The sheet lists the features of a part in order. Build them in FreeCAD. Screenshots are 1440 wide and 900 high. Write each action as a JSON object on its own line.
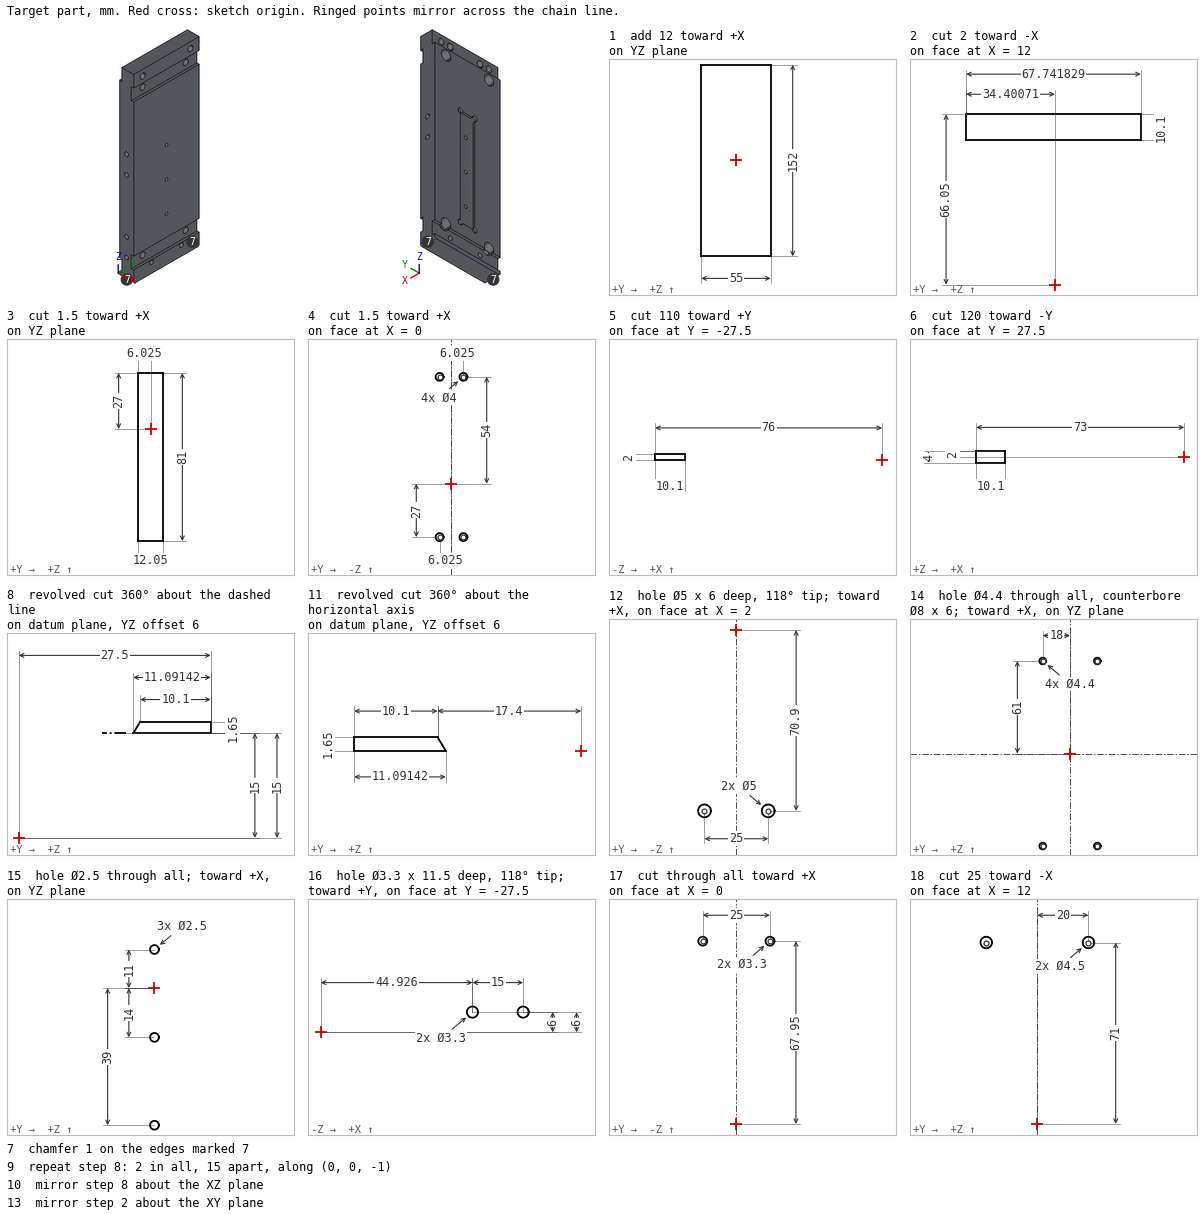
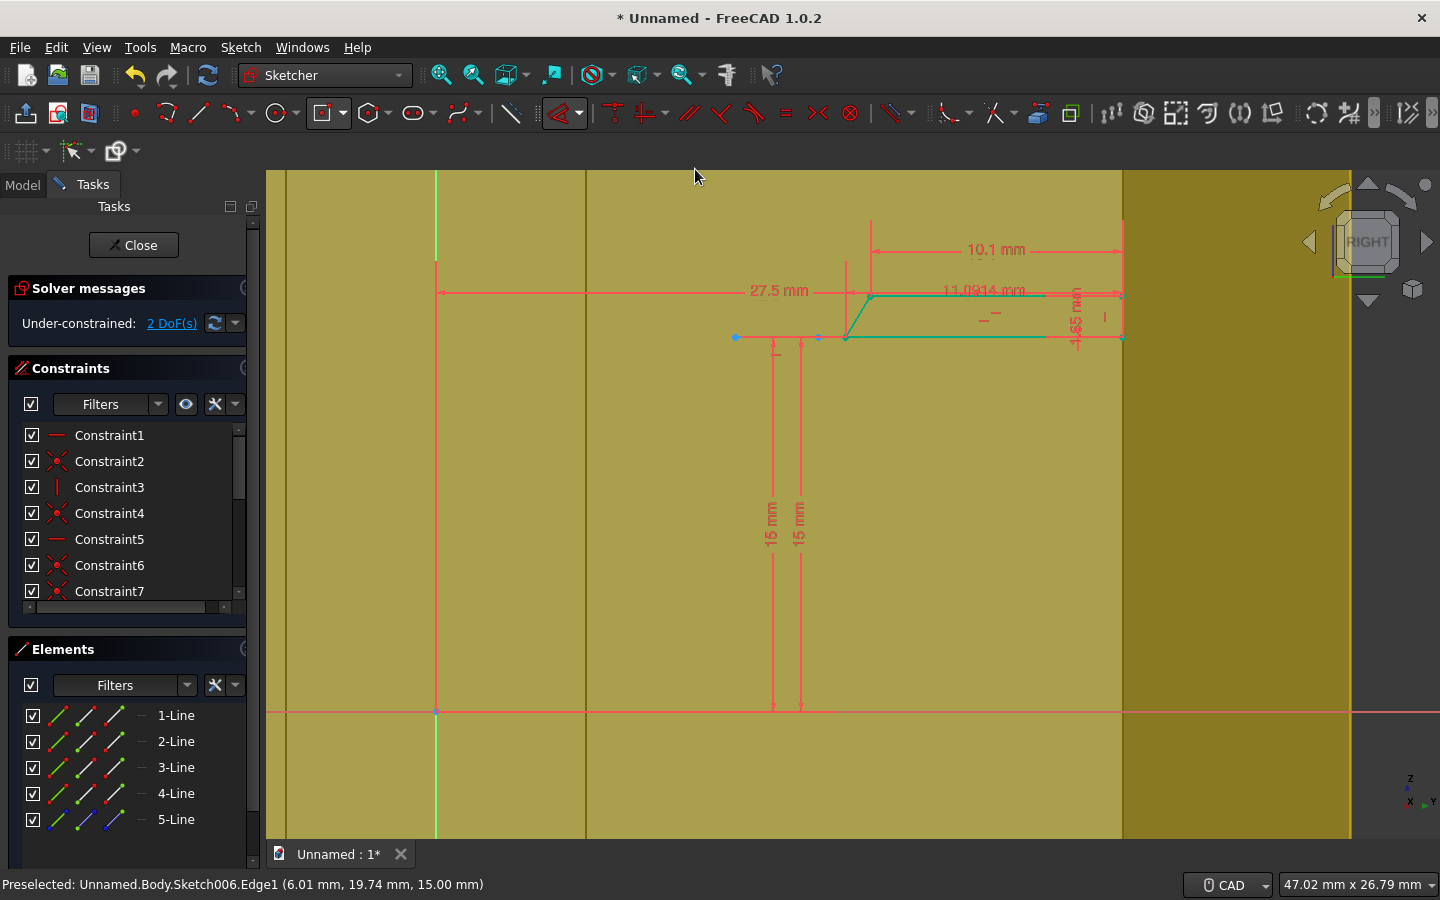
{"action": "left_click", "coordinate": [134, 245]}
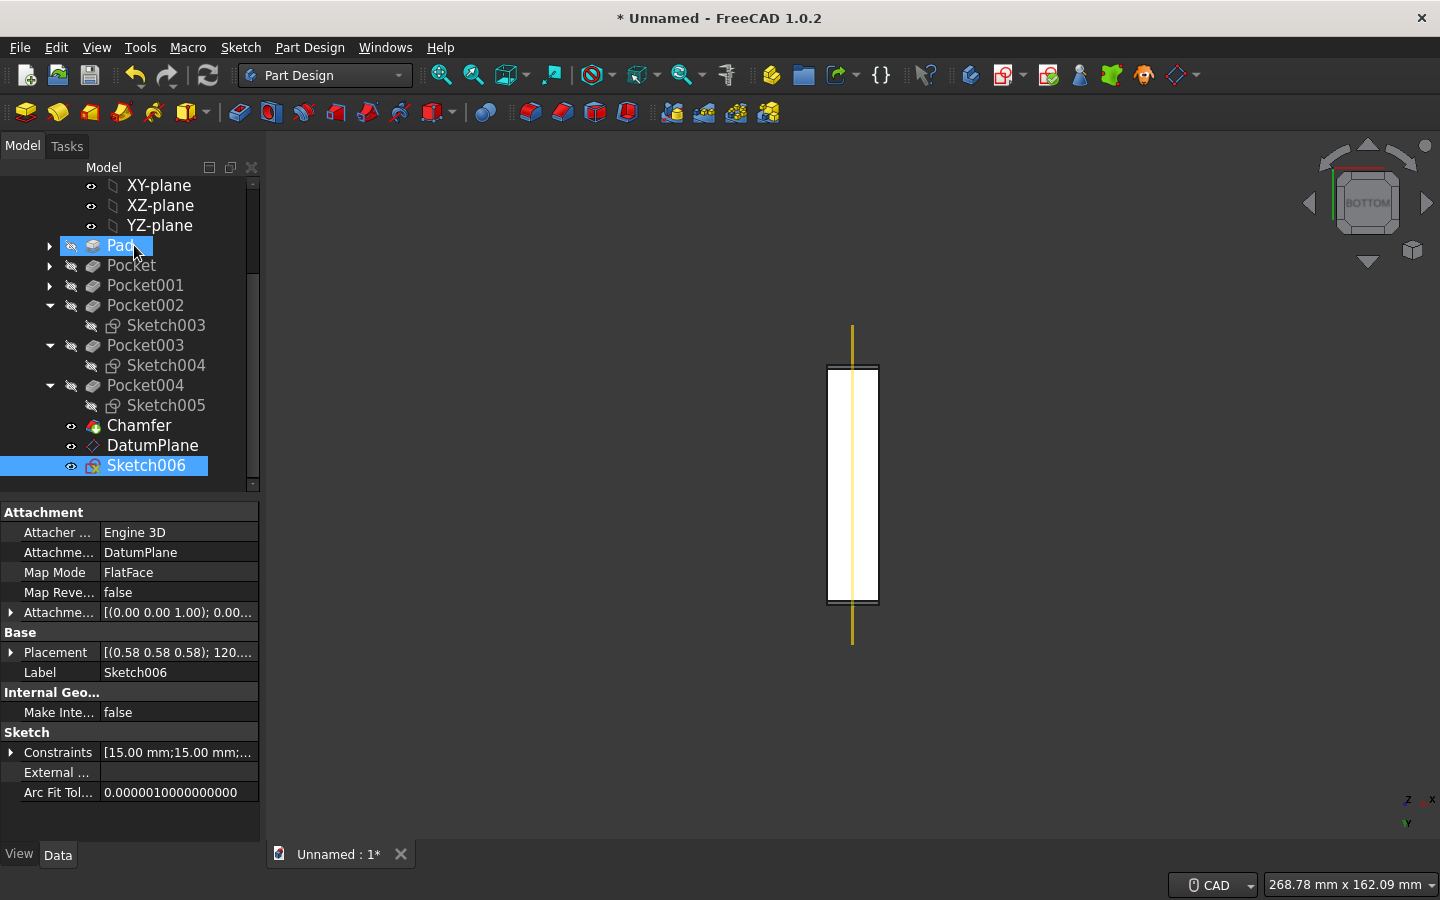
{"action": "left_click", "coordinate": [304, 112]}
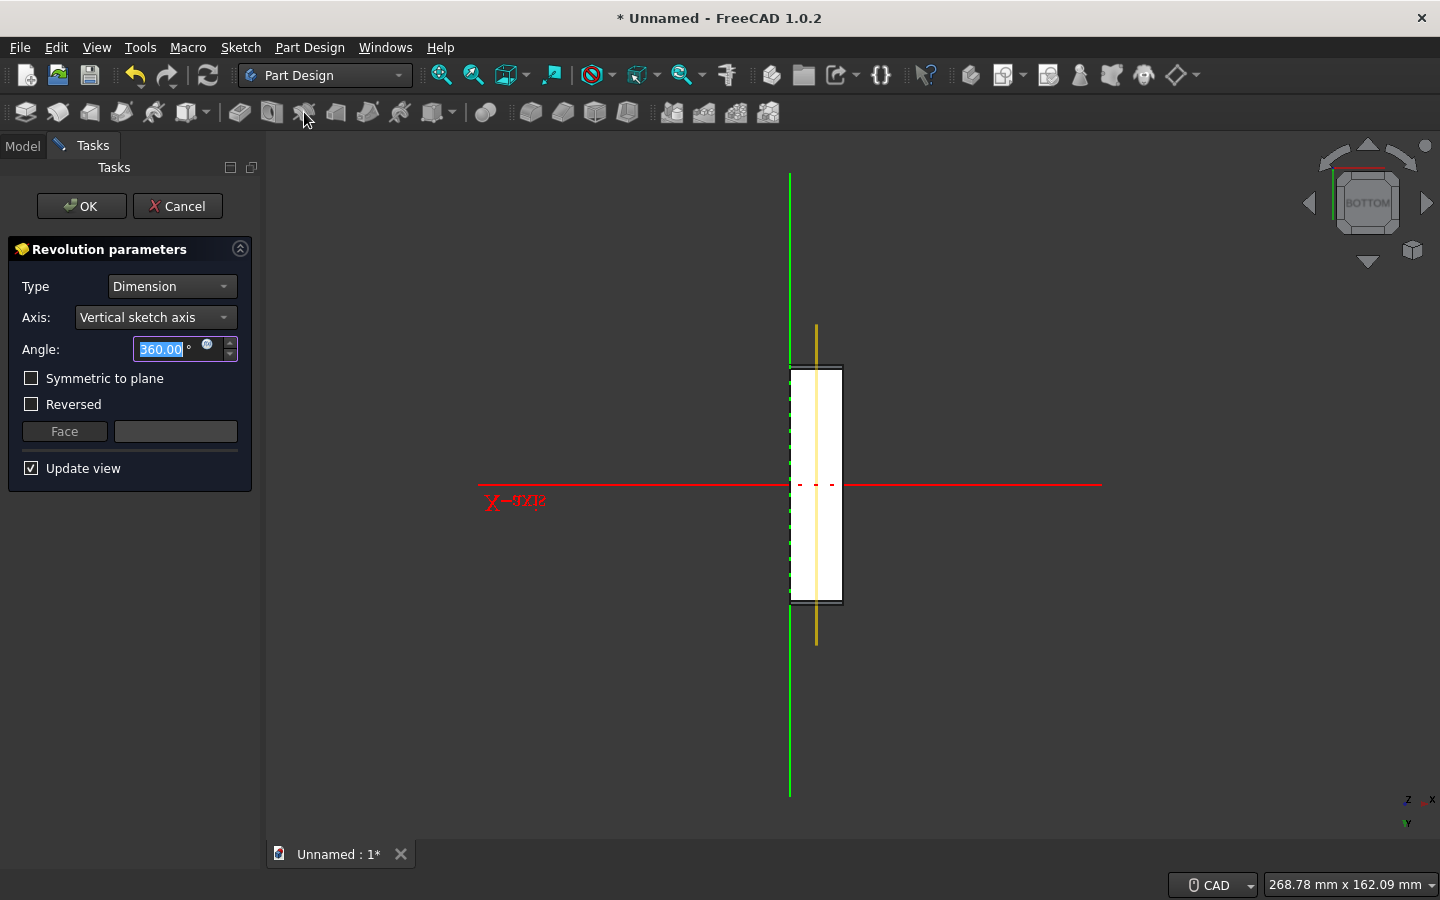
{"action": "left_click", "coordinate": [156, 318]}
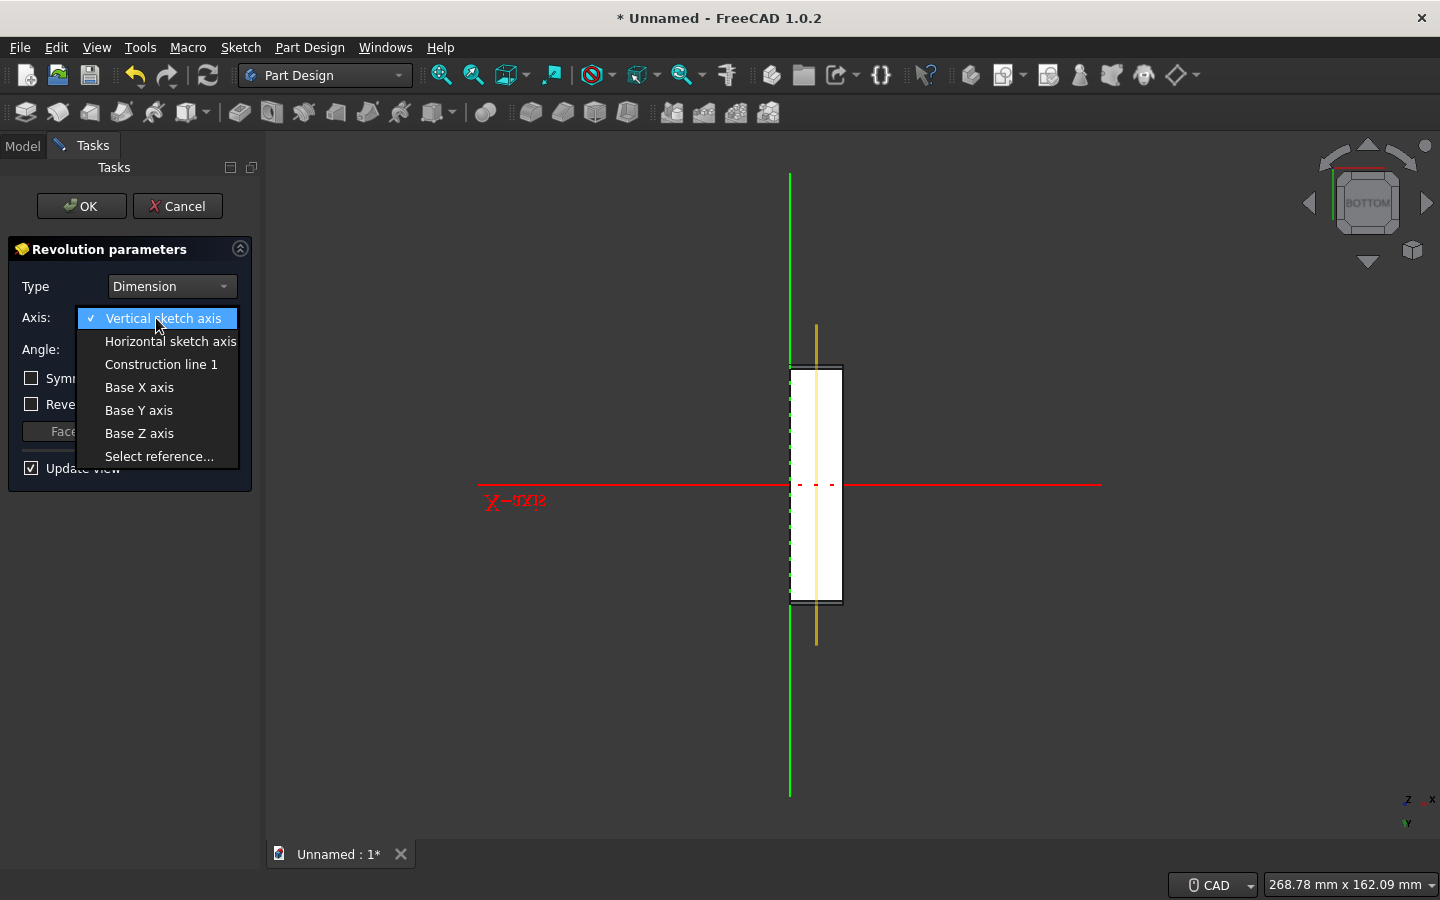
{"action": "left_click", "coordinate": [156, 364]}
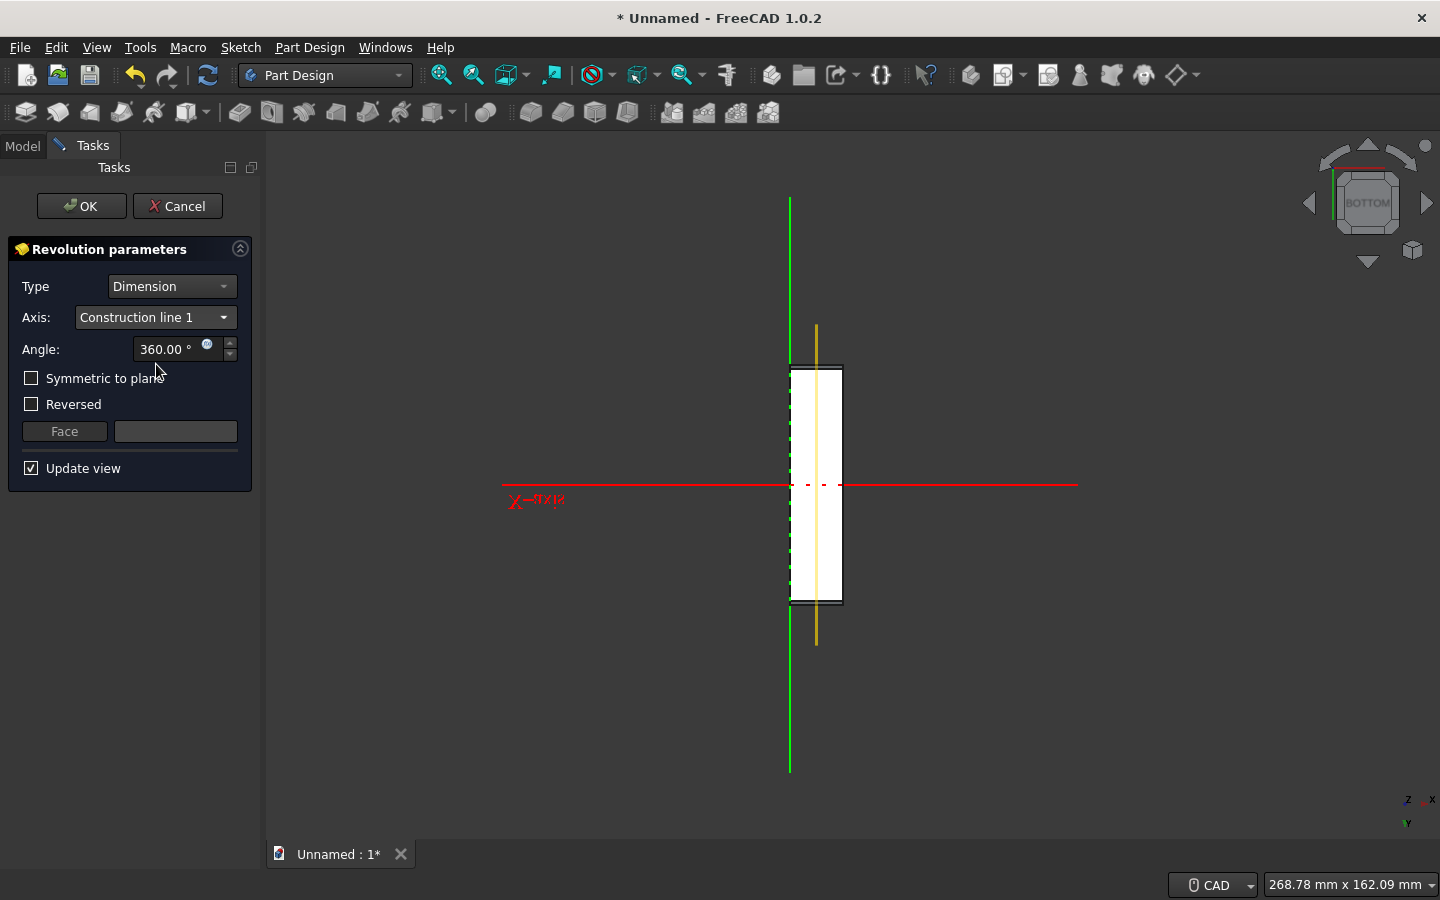
{"action": "left_click", "coordinate": [82, 206]}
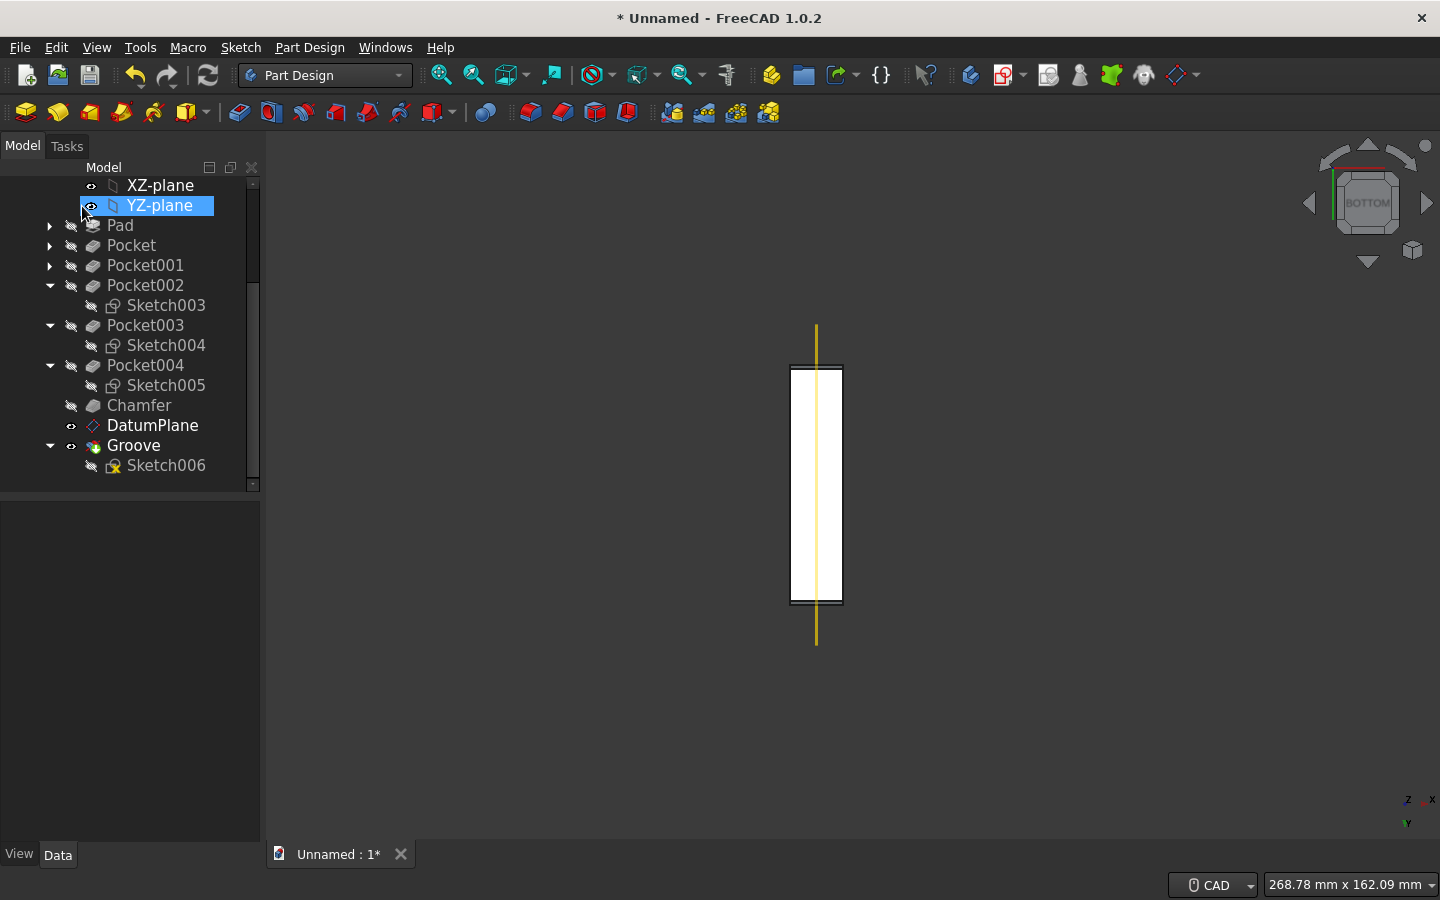
{"action": "left_click", "coordinate": [116, 426]}
{"action": "key", "text": "space"}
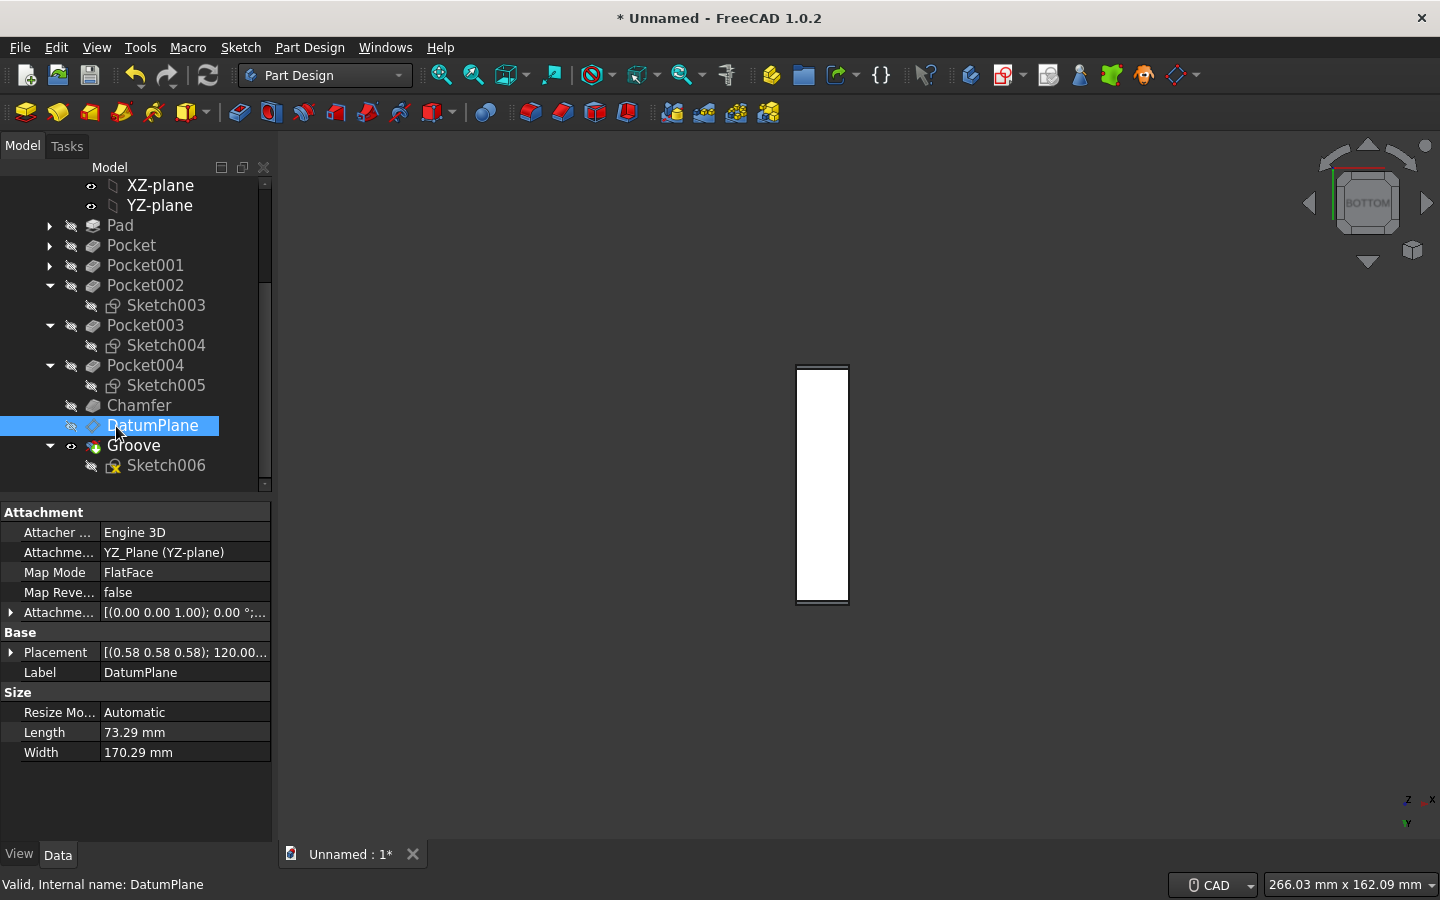
{"action": "key", "text": "v f"}